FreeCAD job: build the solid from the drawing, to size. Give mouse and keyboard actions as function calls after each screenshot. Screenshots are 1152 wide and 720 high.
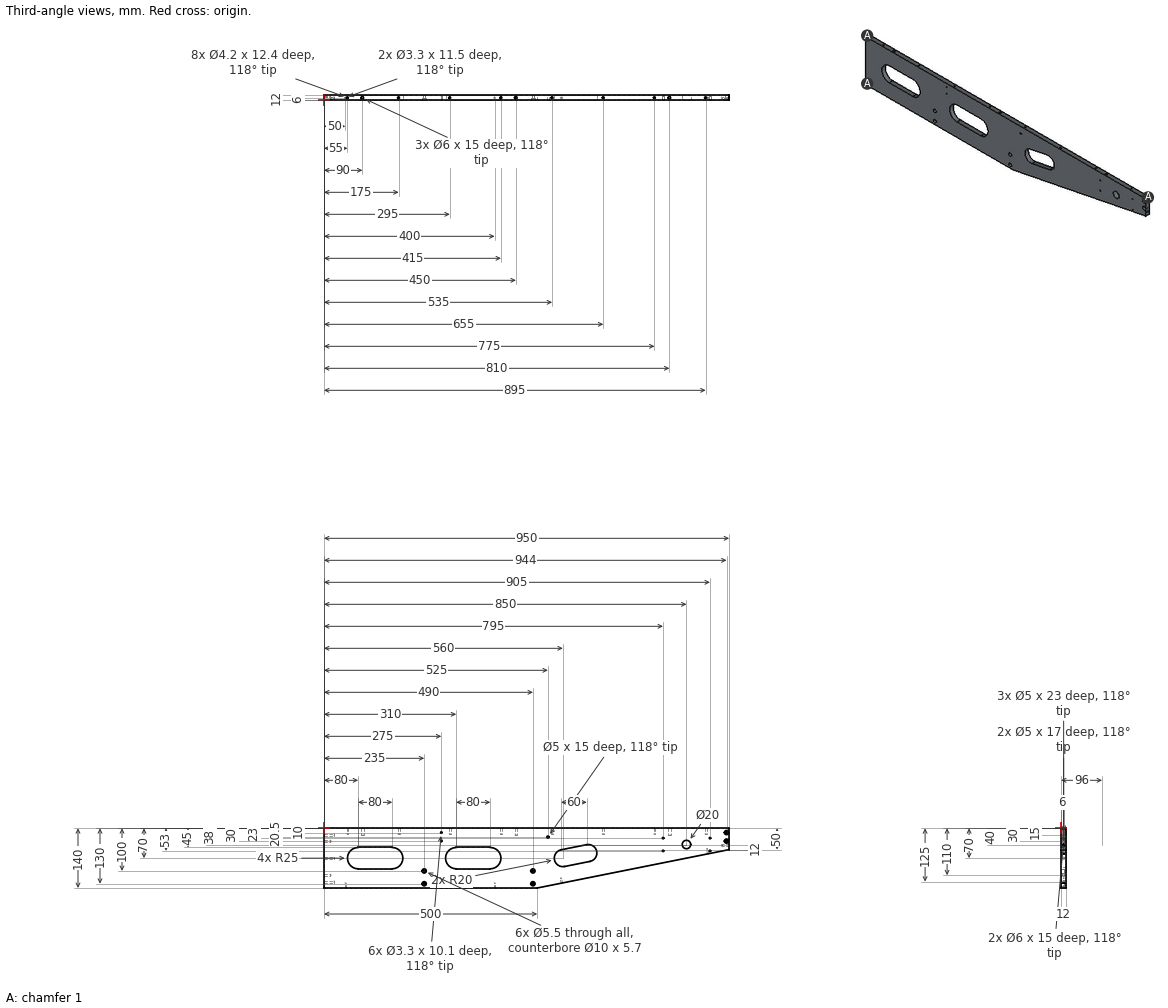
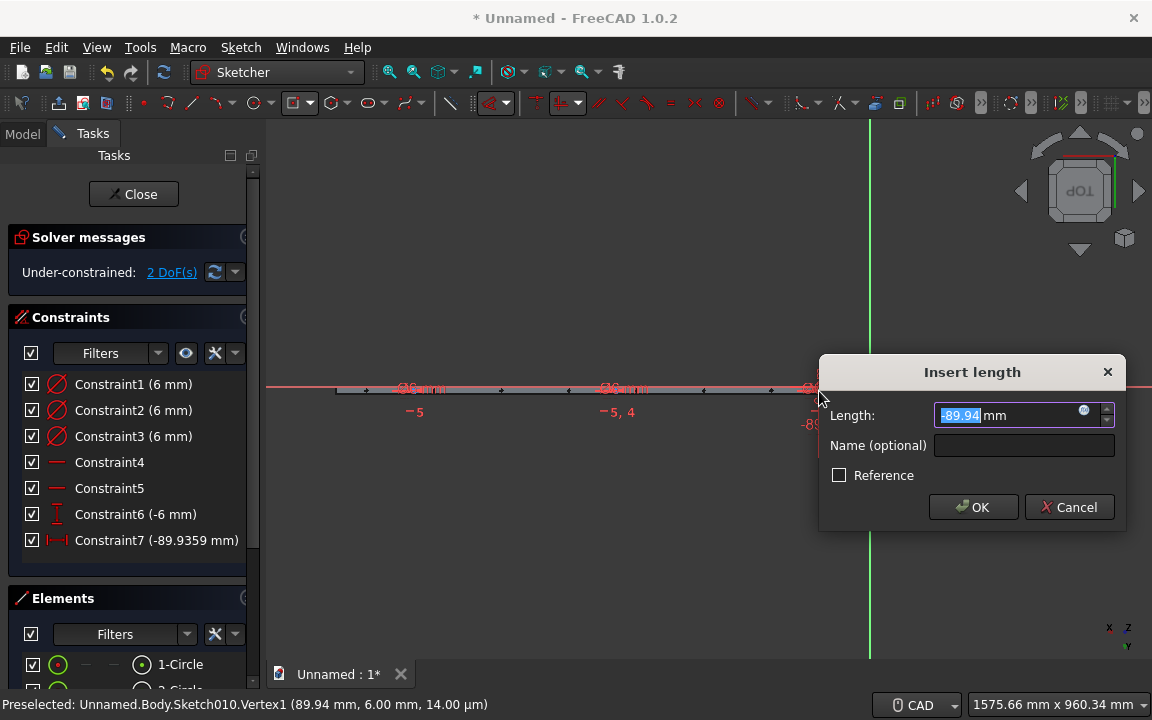
text(-90)
key(Return)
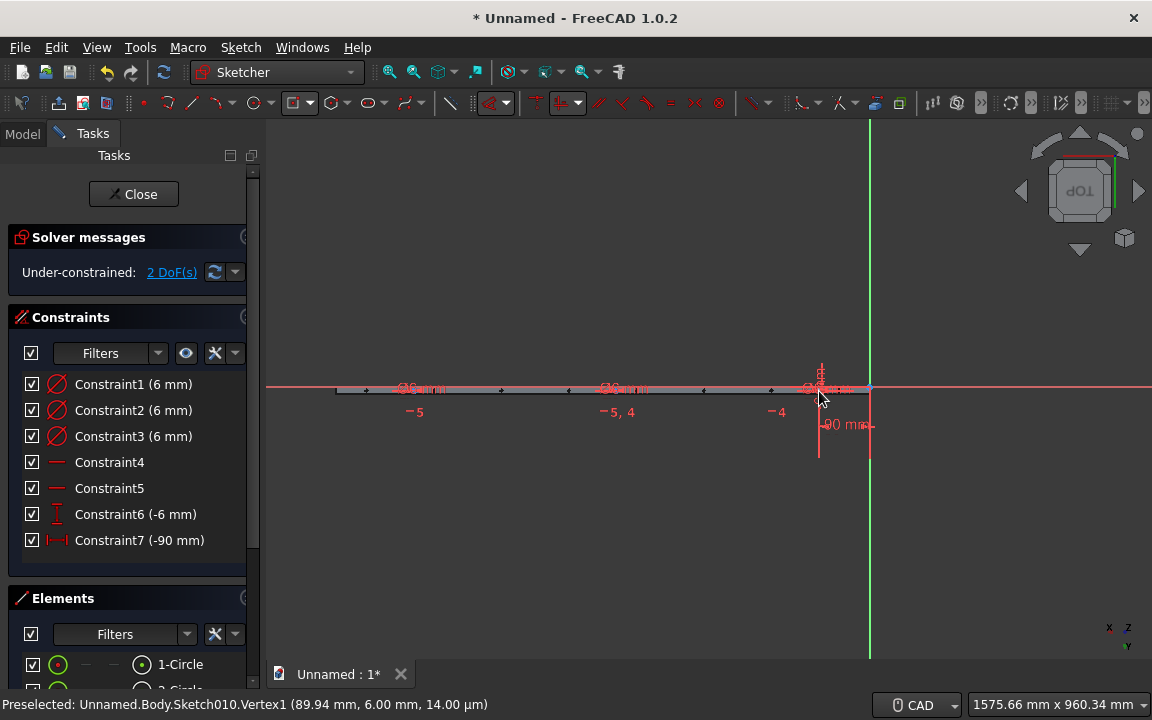
click(617, 391)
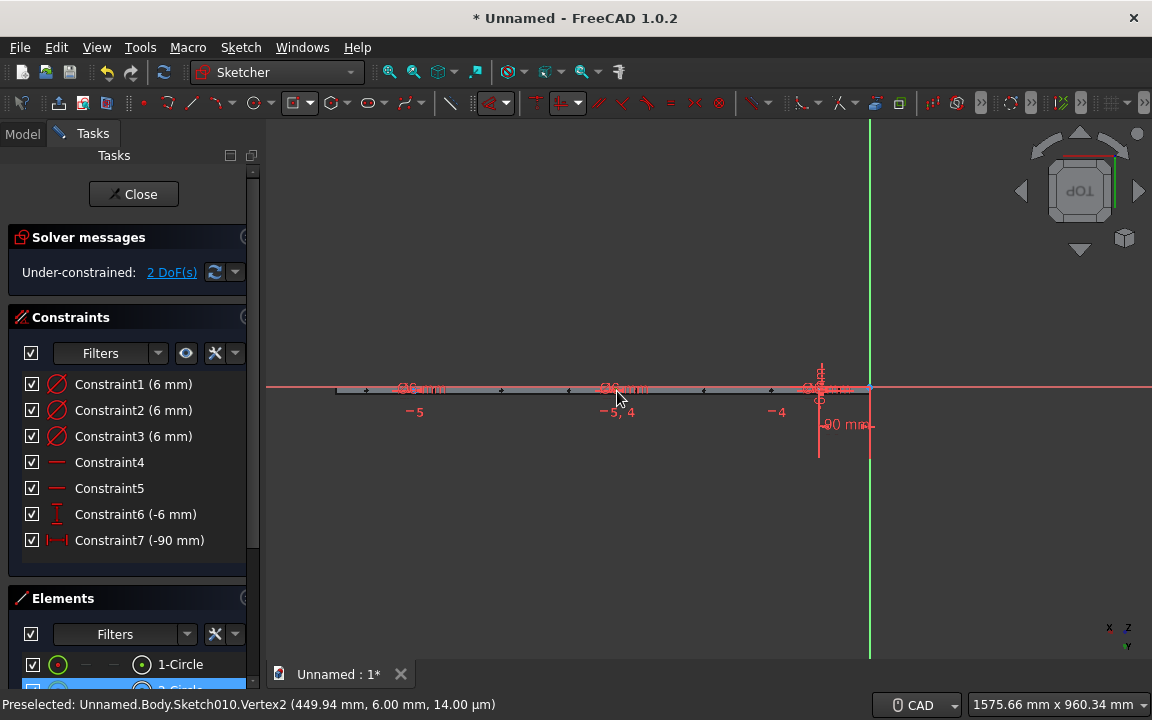
key(l)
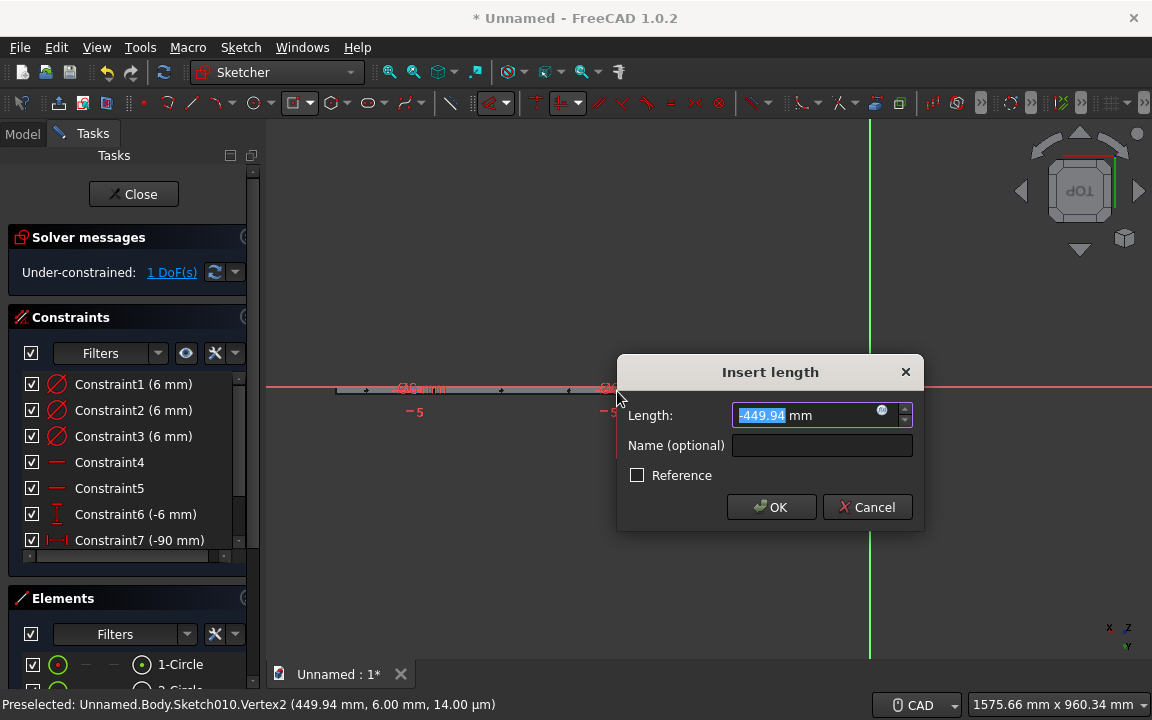
text(-450)
key(Return)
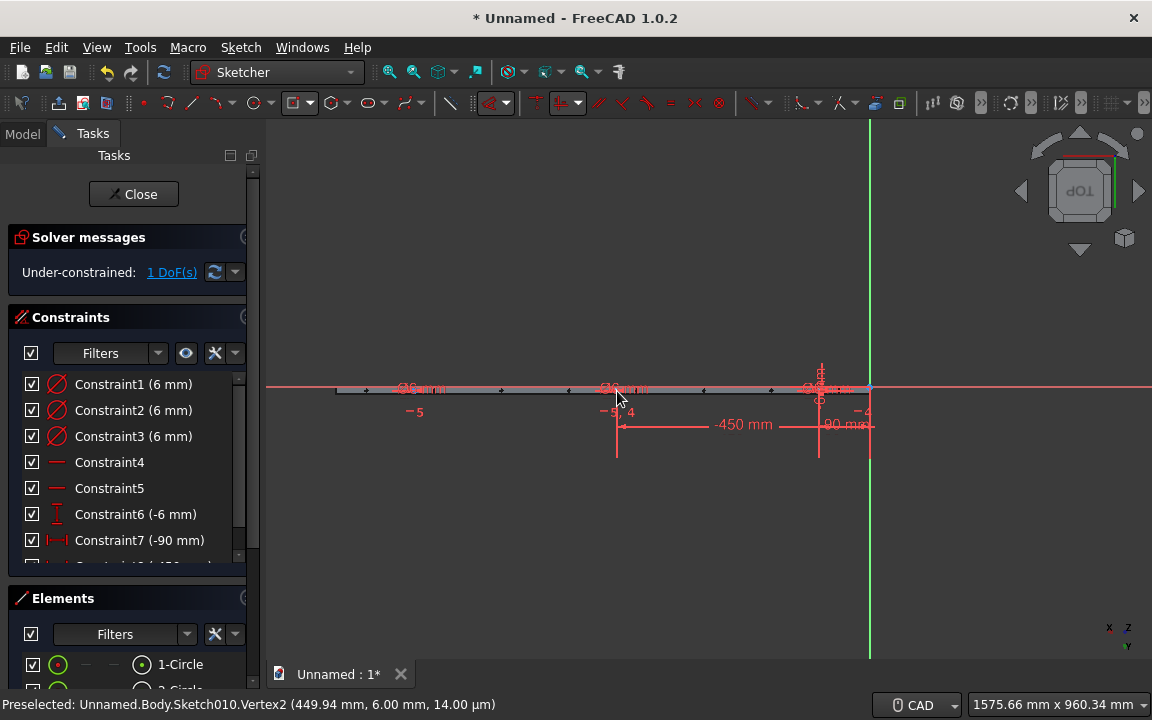
click(414, 391)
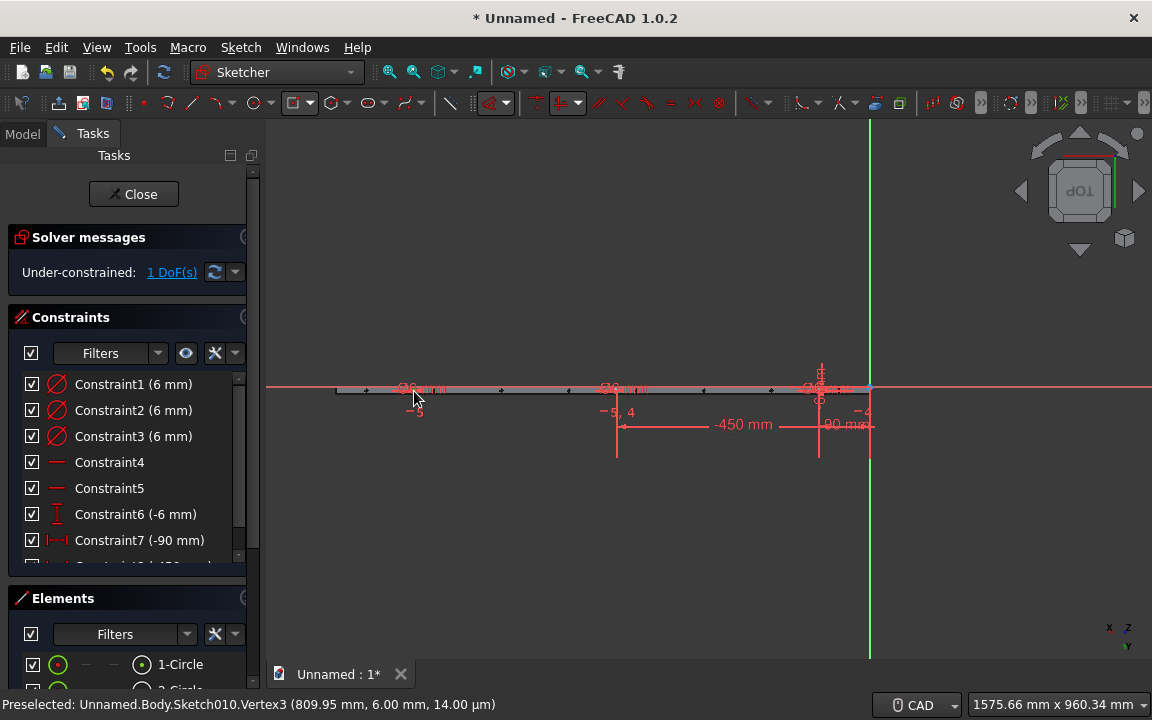
key(l)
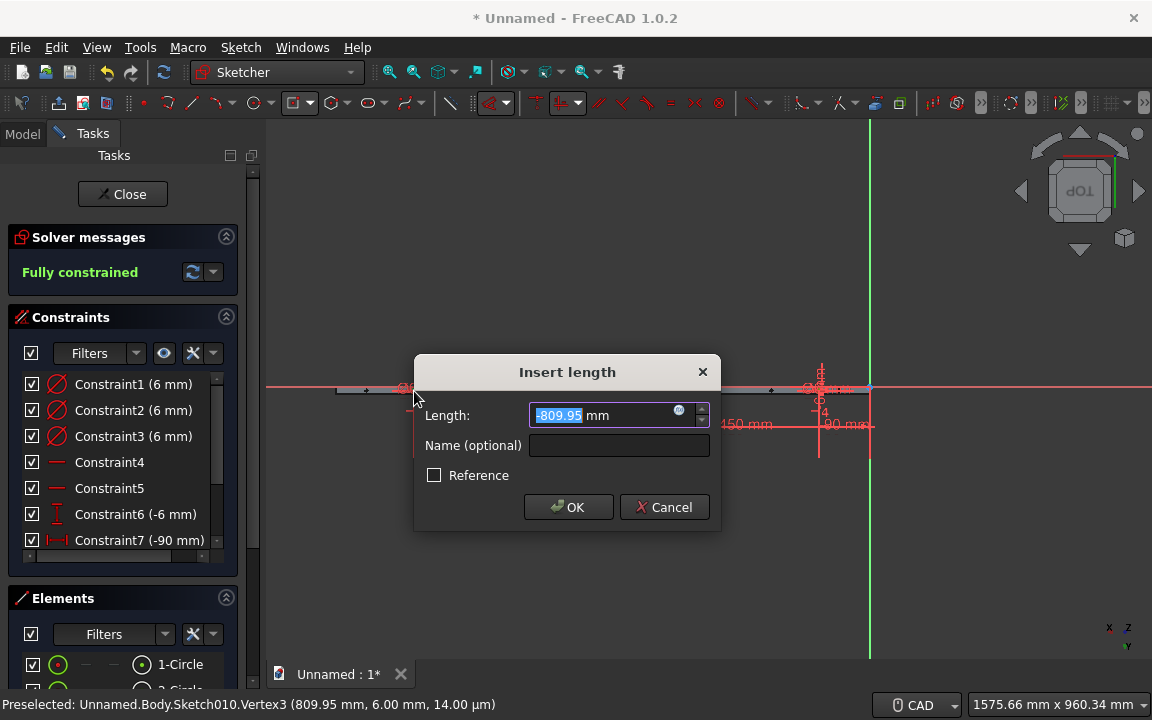
text(-810)
key(Return)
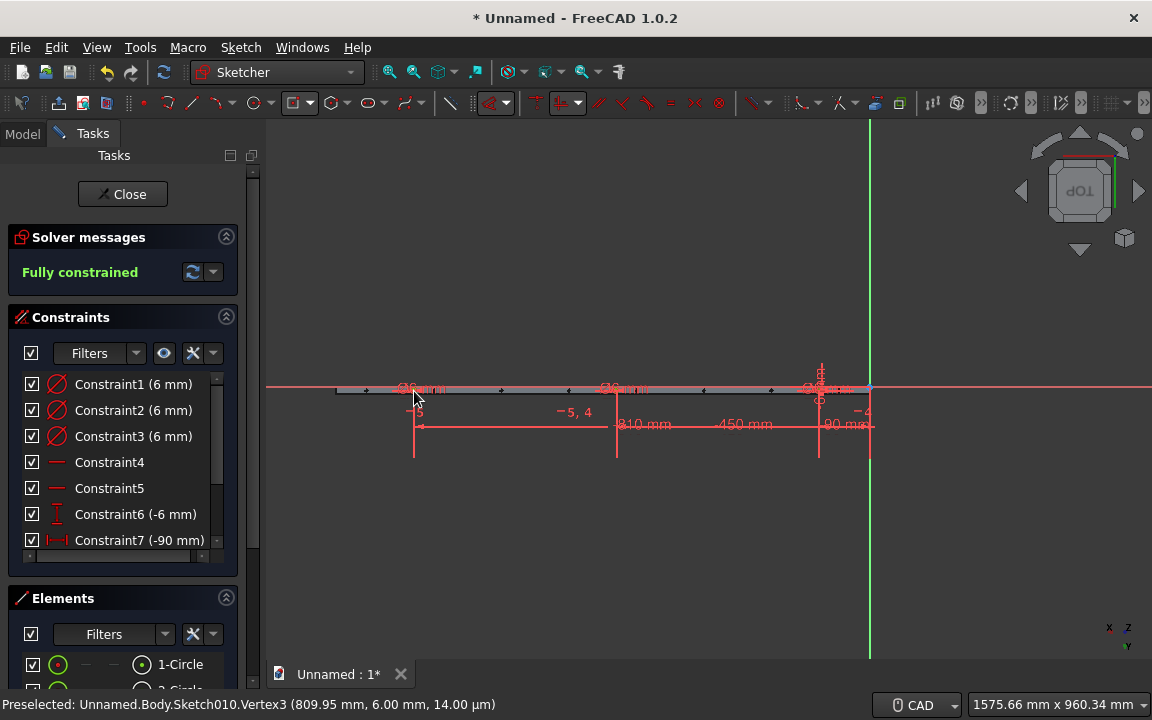
click(123, 194)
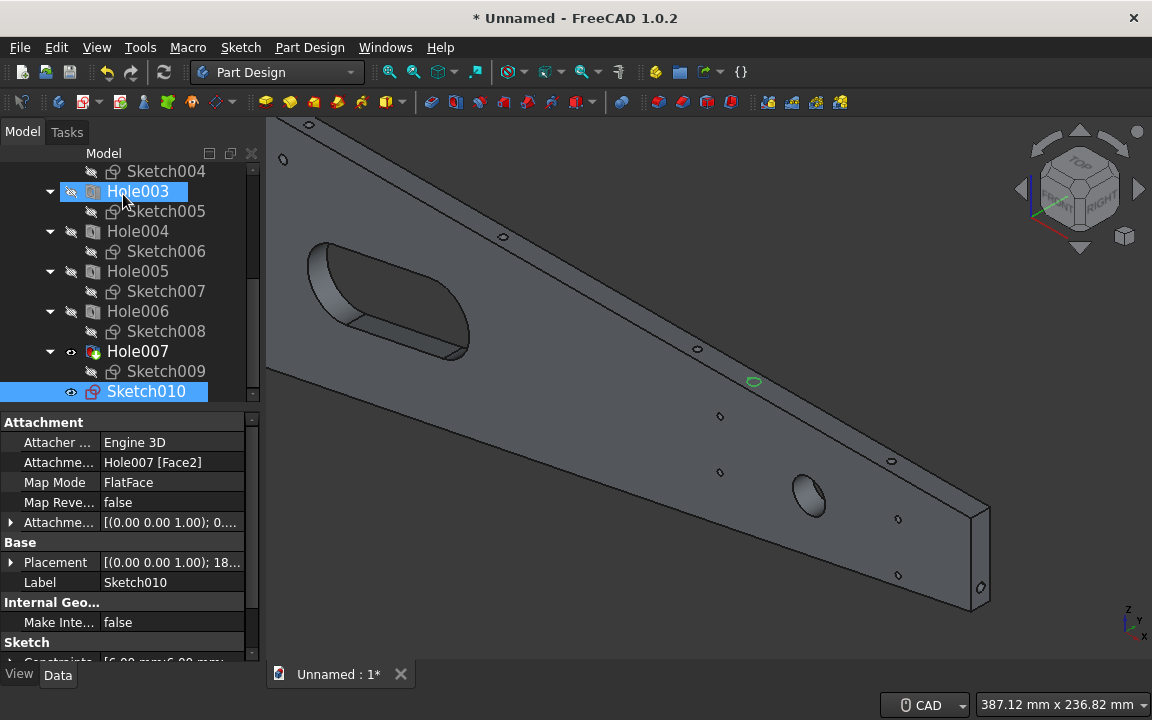
click(456, 102)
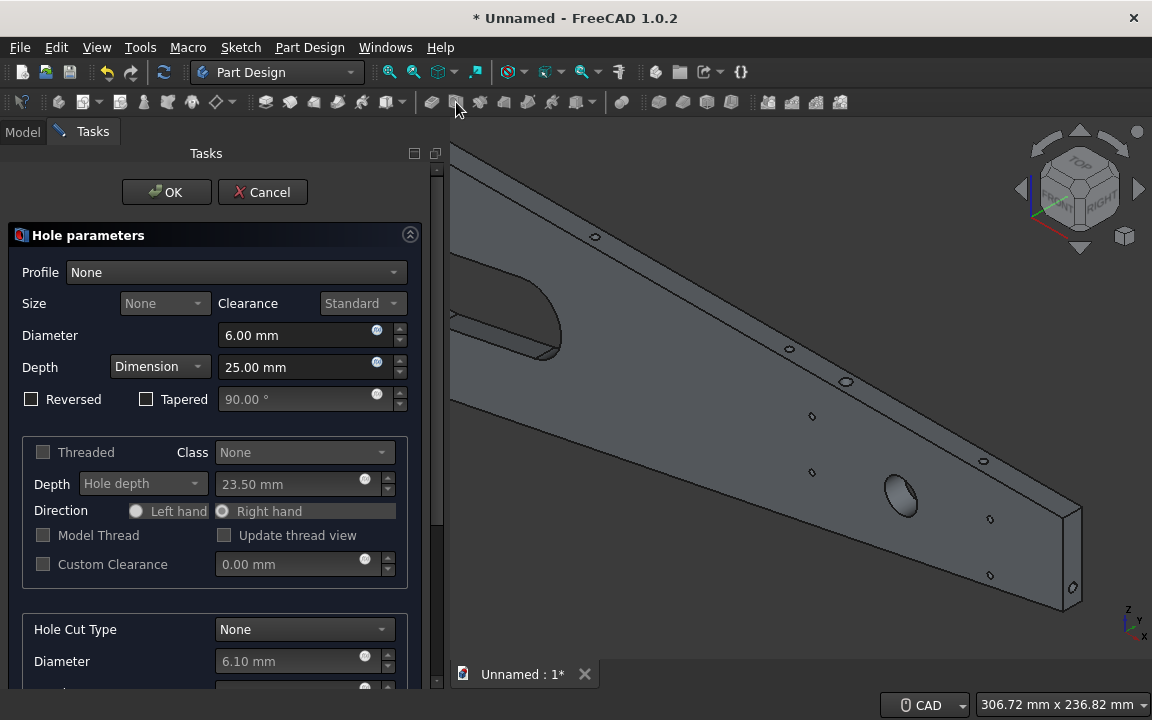
triple_click(305, 335)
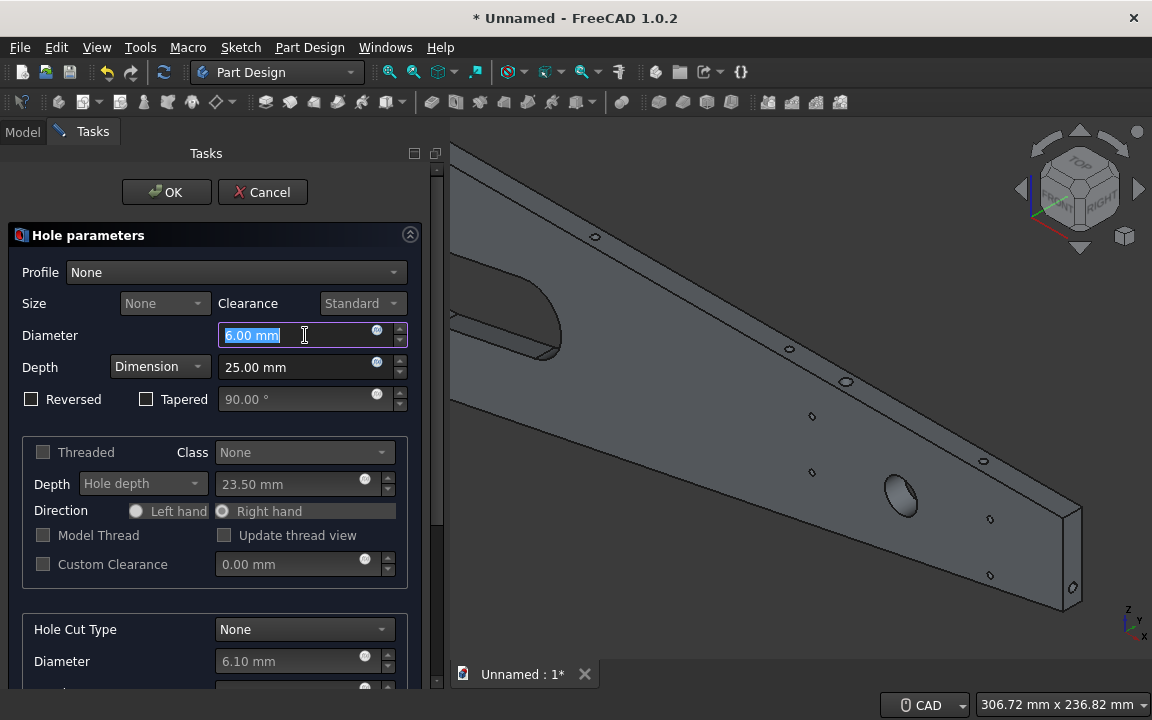
text(6)
key(Tab)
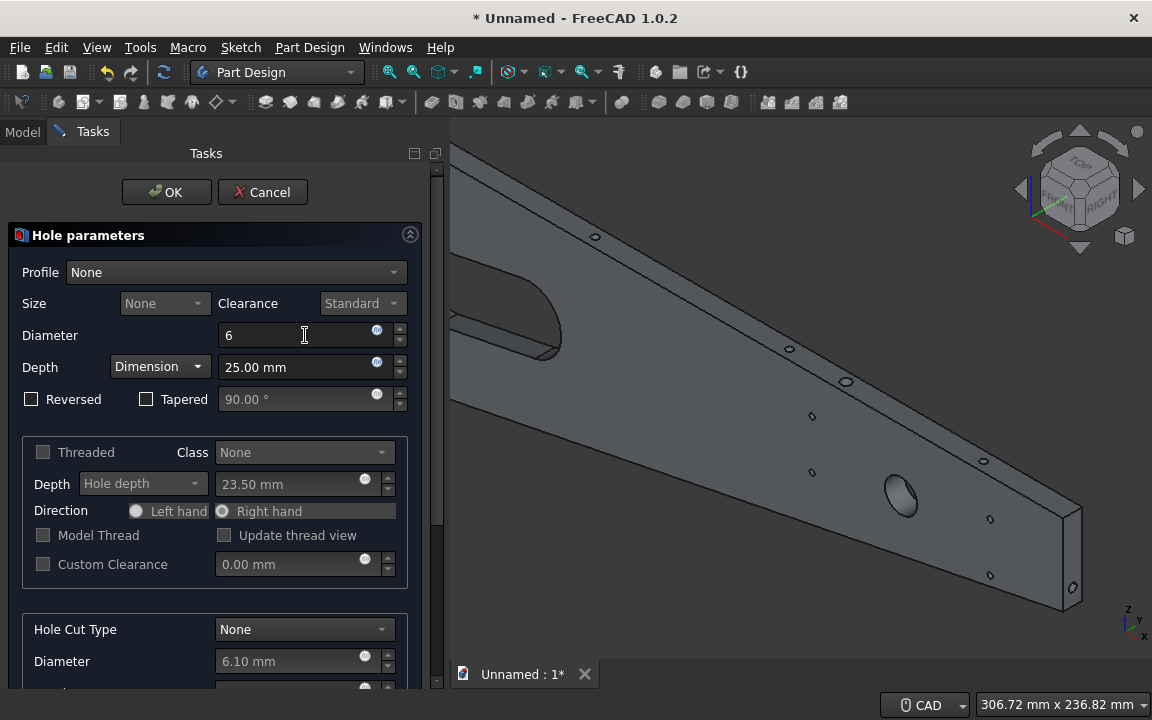
triple_click(305, 367)